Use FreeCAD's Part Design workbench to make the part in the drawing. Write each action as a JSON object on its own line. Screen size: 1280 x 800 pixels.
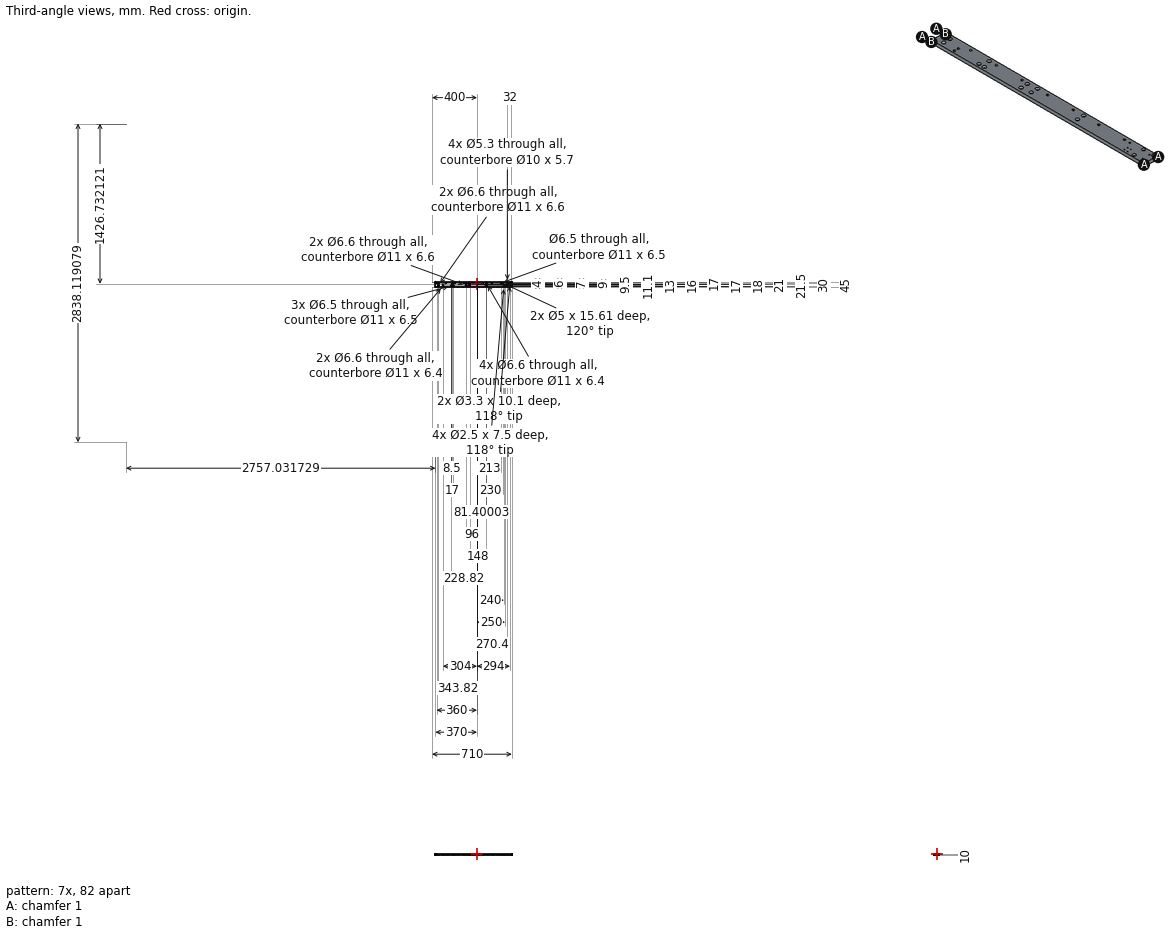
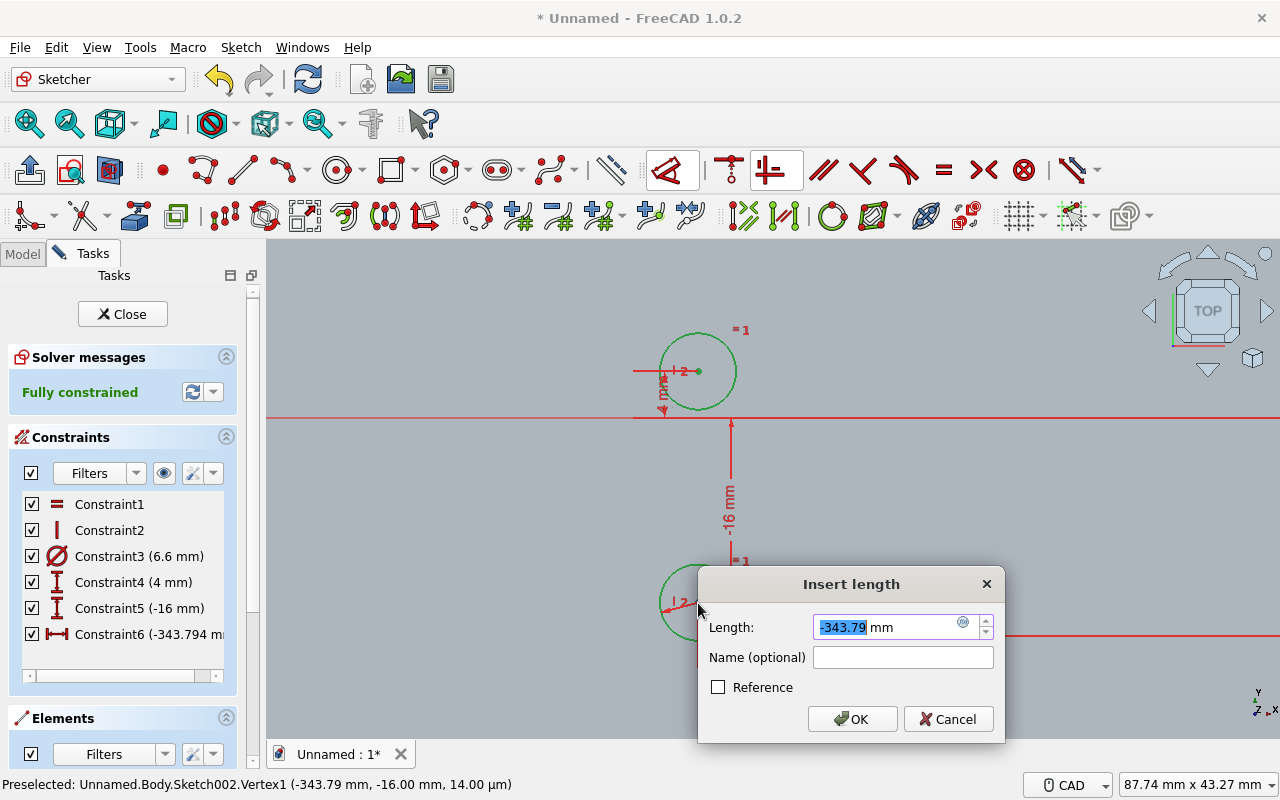
{"action": "type", "text": "-343.82"}
{"action": "key", "text": "Return"}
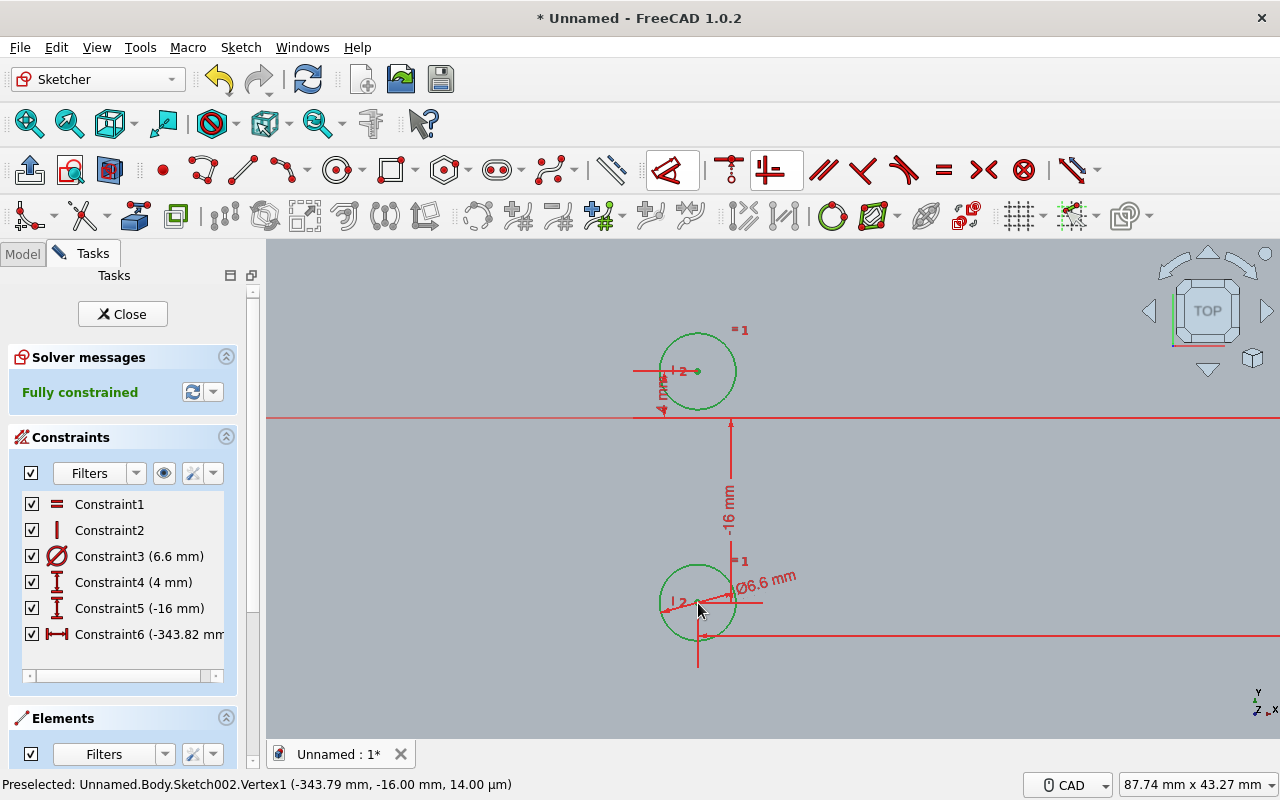
{"action": "left_click", "coordinate": [123, 314]}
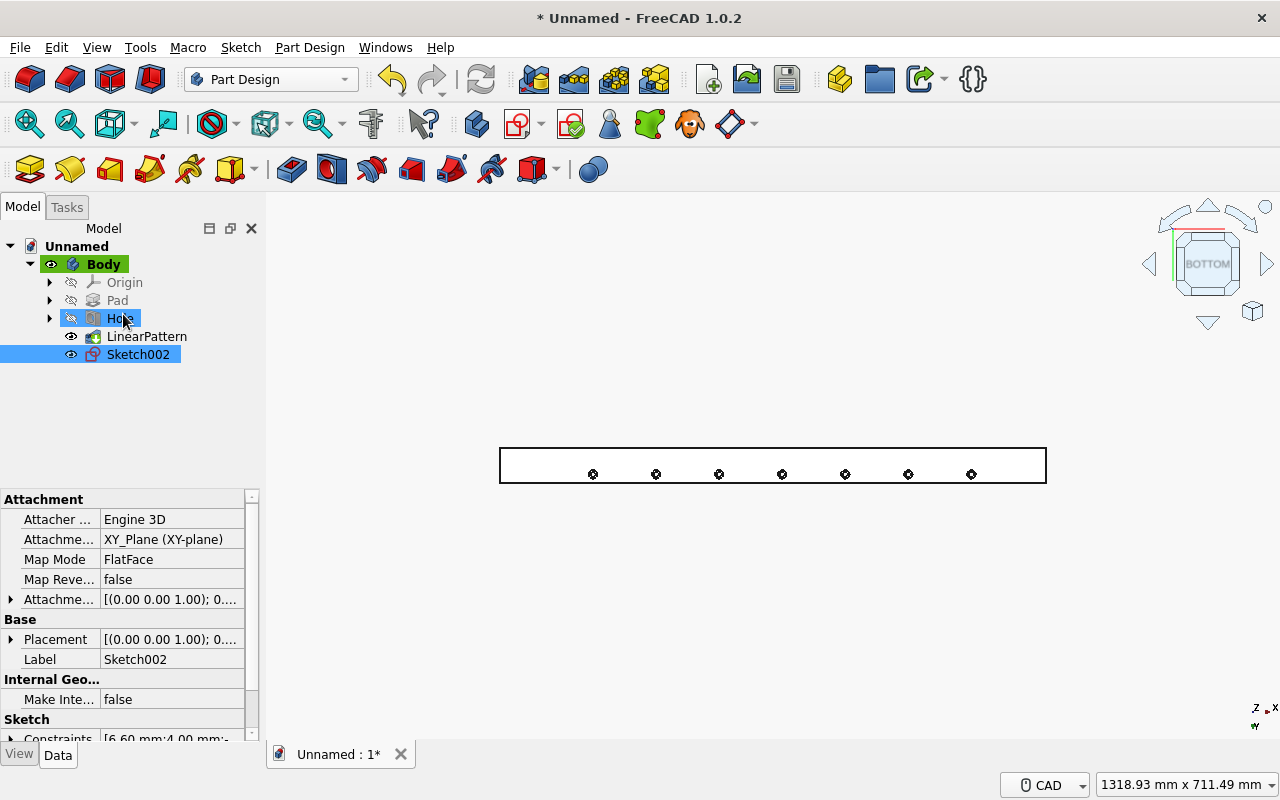
{"action": "left_click", "coordinate": [332, 170]}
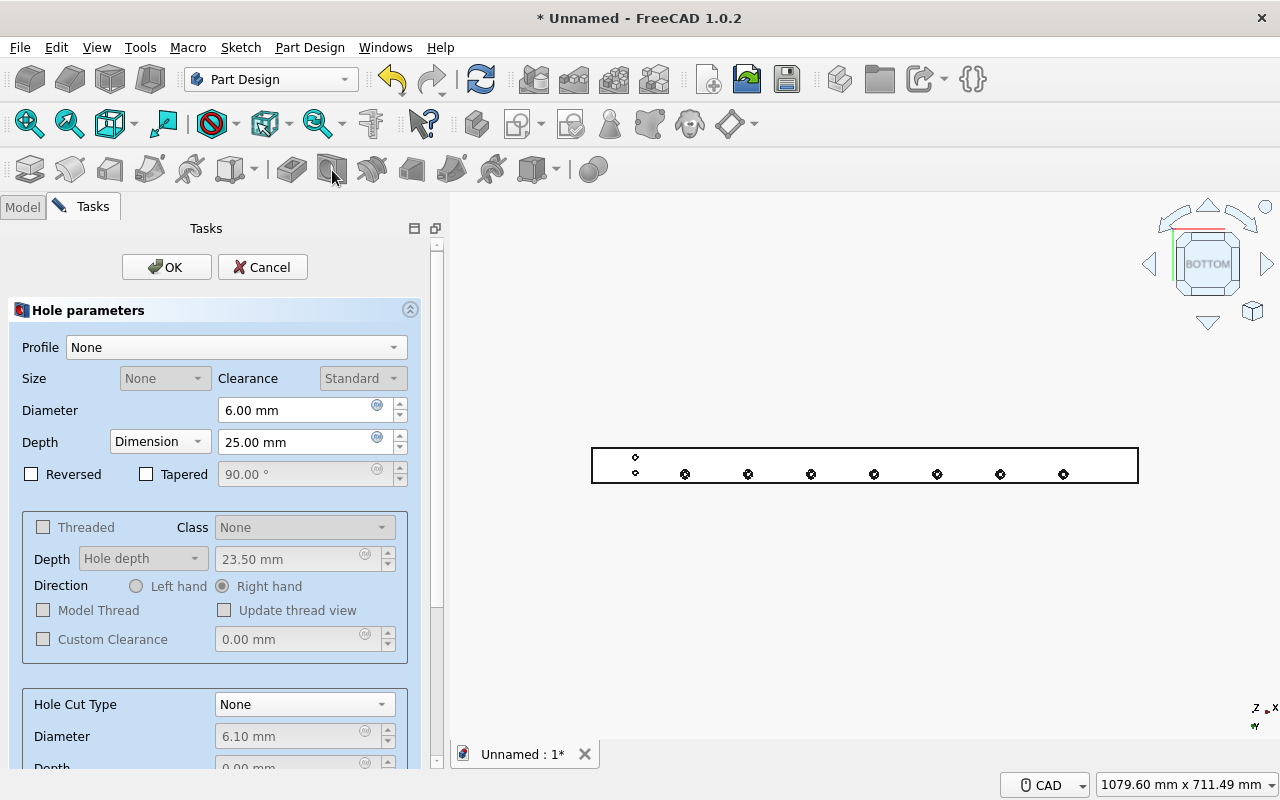
{"action": "triple_click", "coordinate": [305, 410]}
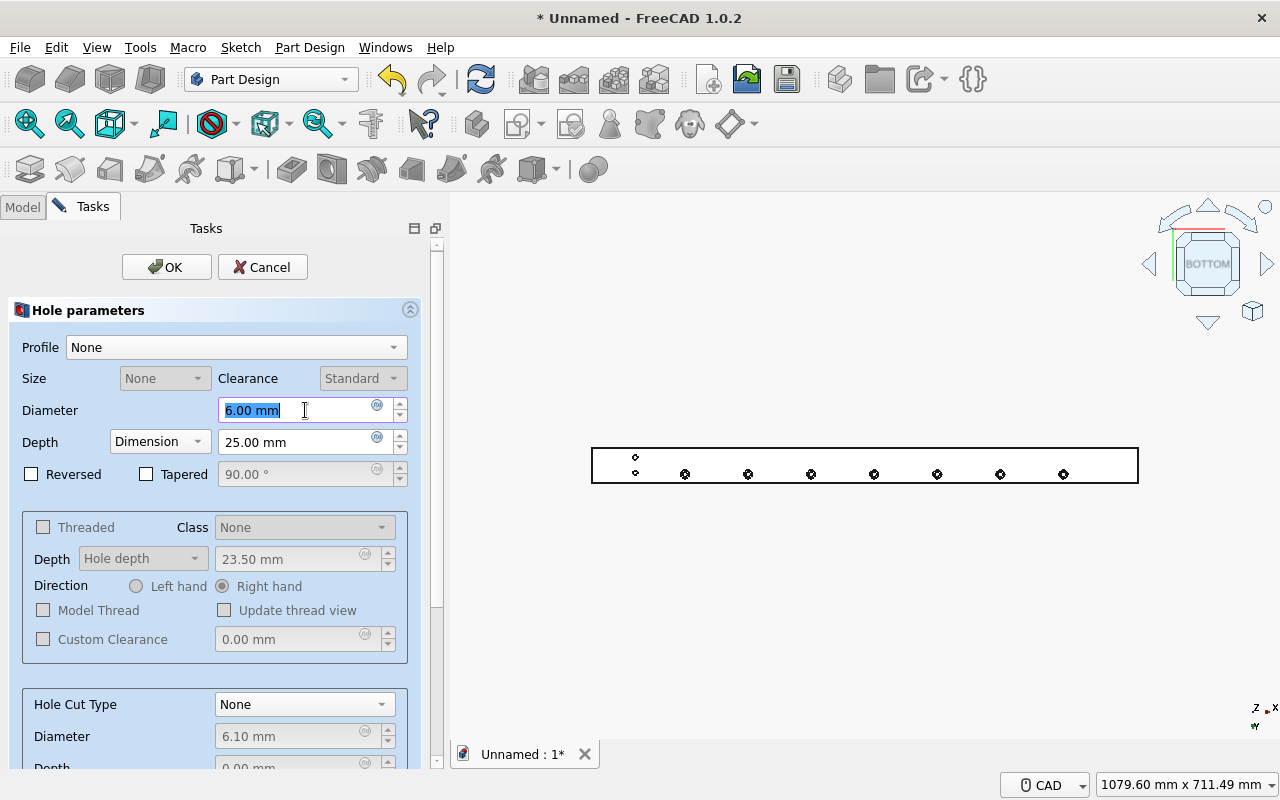
{"action": "type", "text": "6.6"}
{"action": "key", "text": "Tab"}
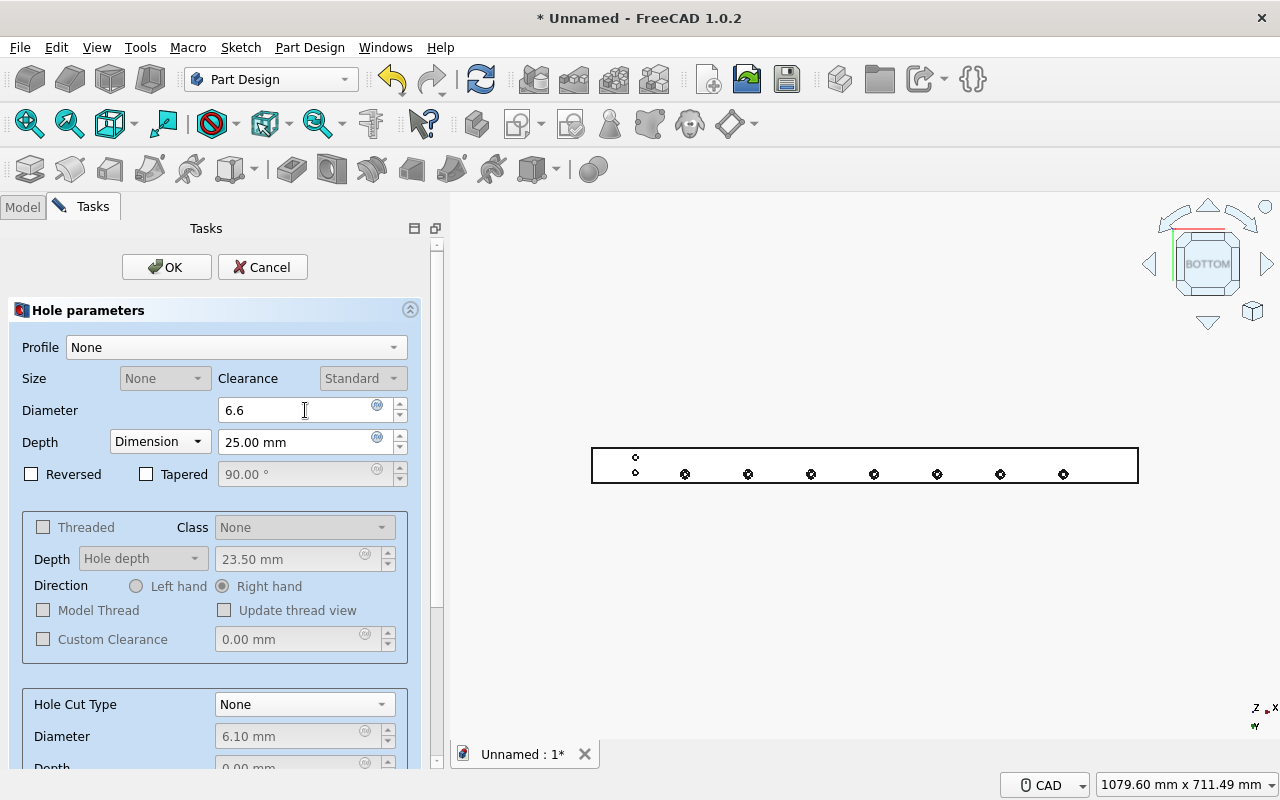
{"action": "left_click", "coordinate": [161, 442]}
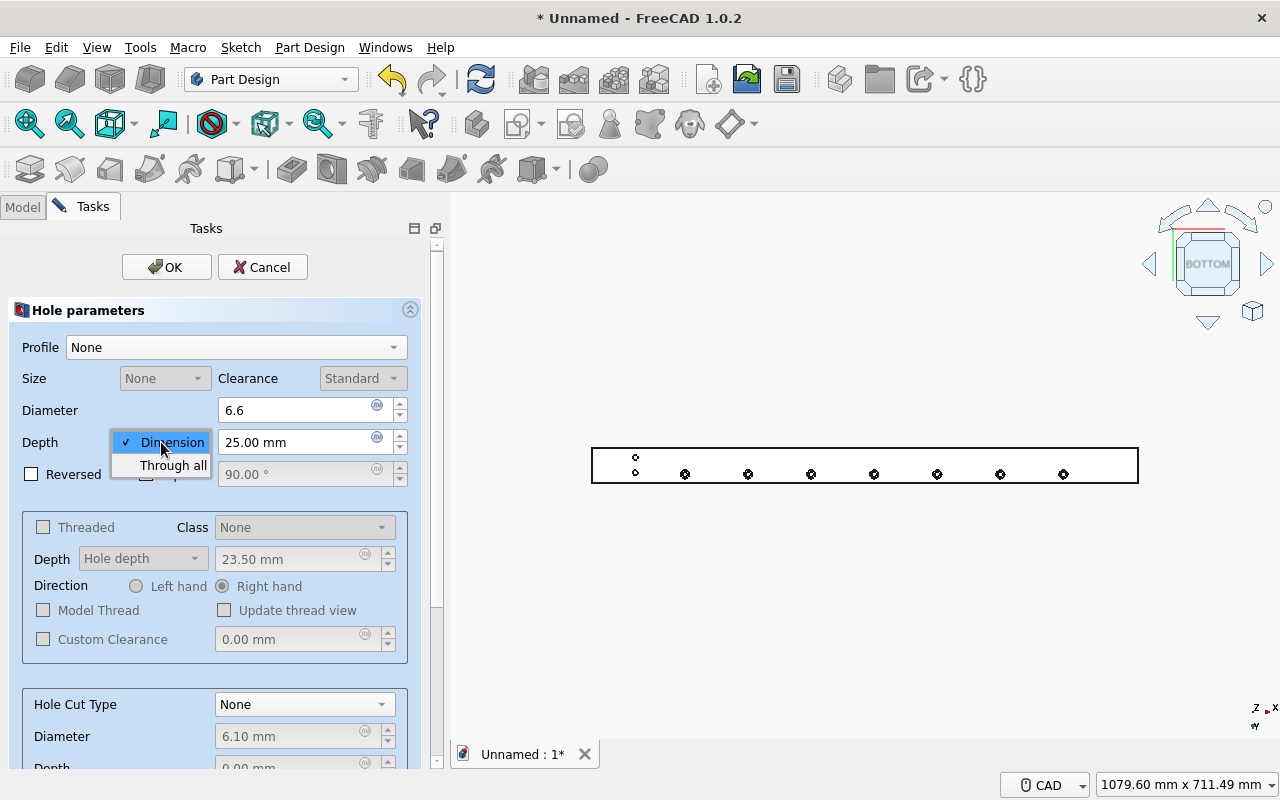
{"action": "left_click", "coordinate": [160, 466]}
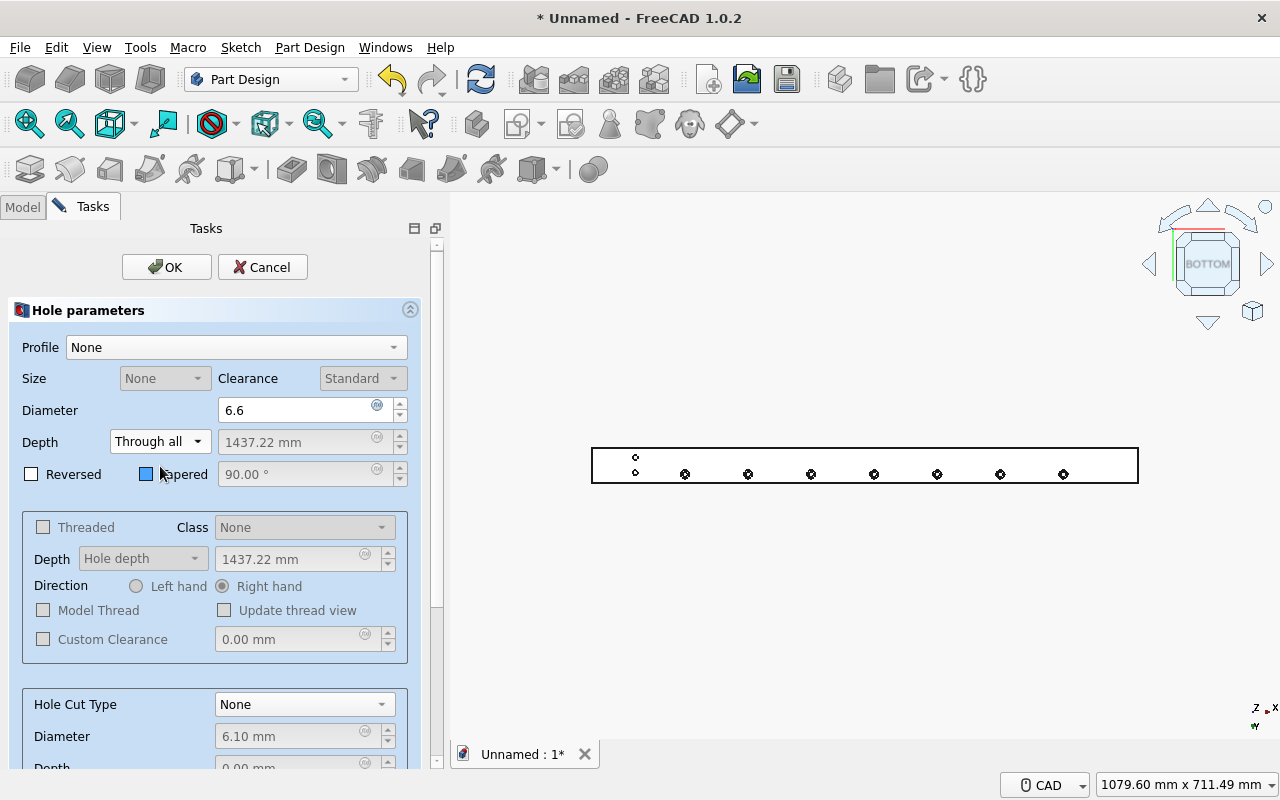
{"action": "left_click", "coordinate": [306, 704]}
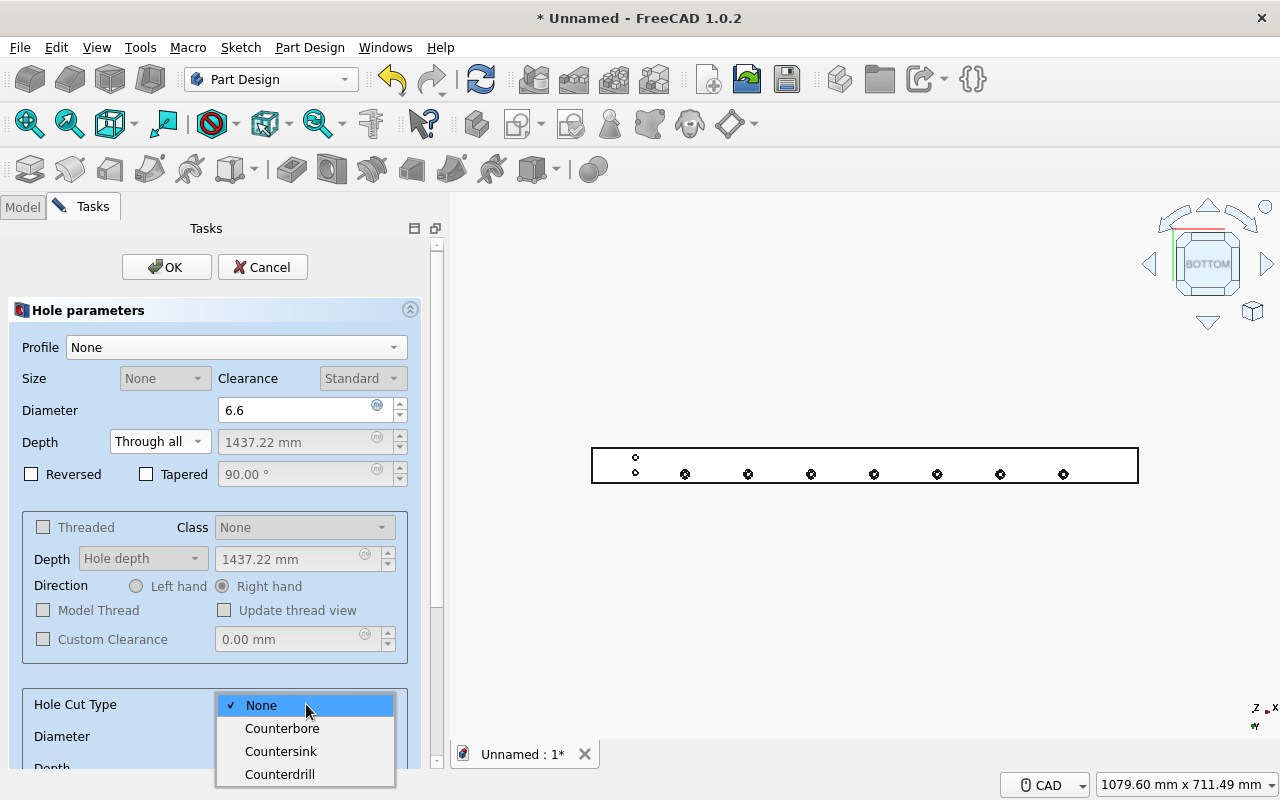
{"action": "left_click", "coordinate": [304, 728]}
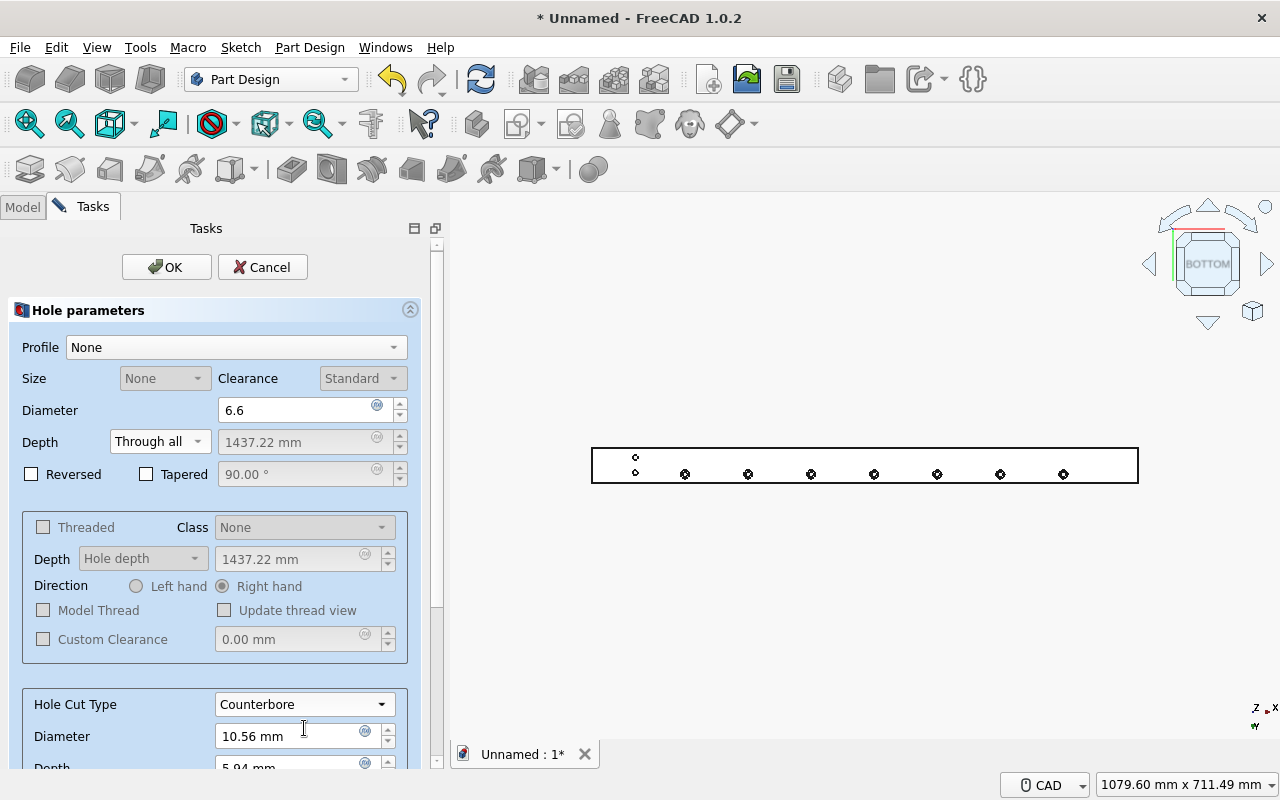
{"action": "triple_click", "coordinate": [298, 736]}